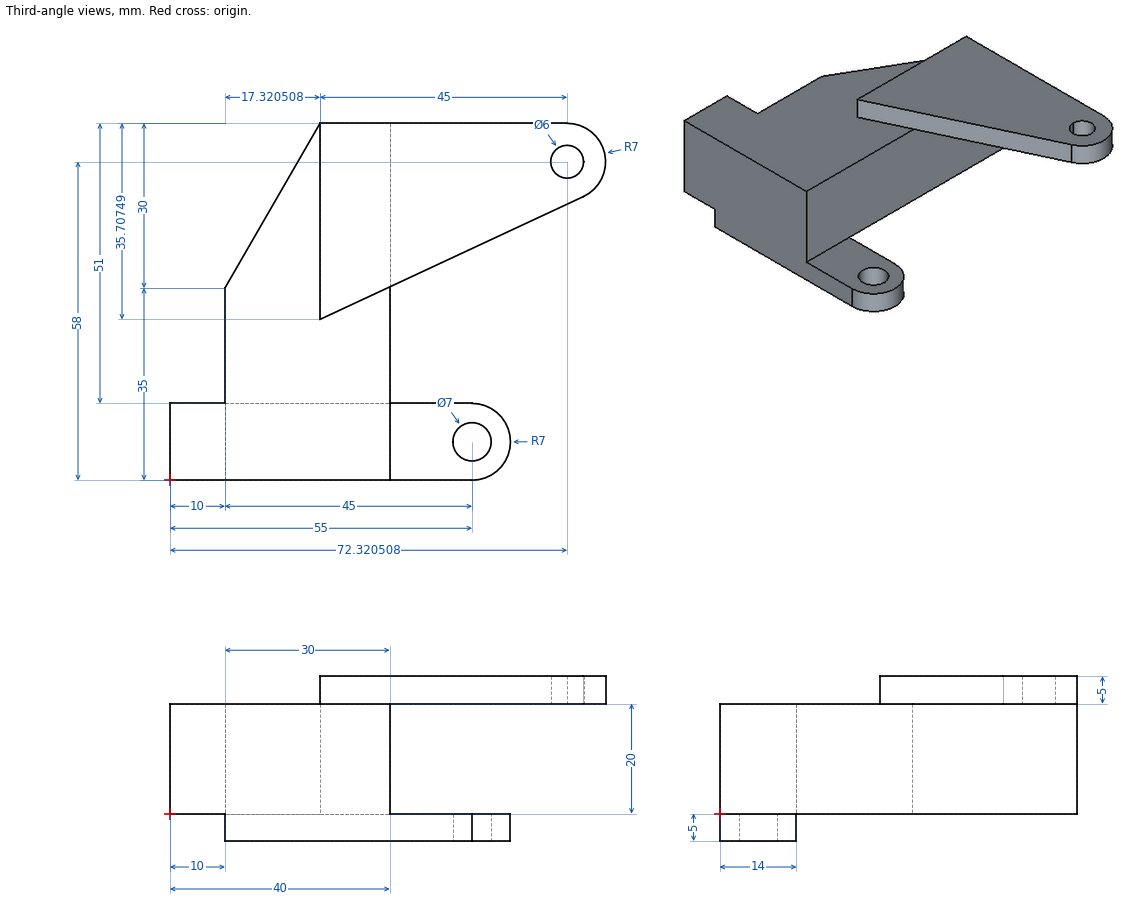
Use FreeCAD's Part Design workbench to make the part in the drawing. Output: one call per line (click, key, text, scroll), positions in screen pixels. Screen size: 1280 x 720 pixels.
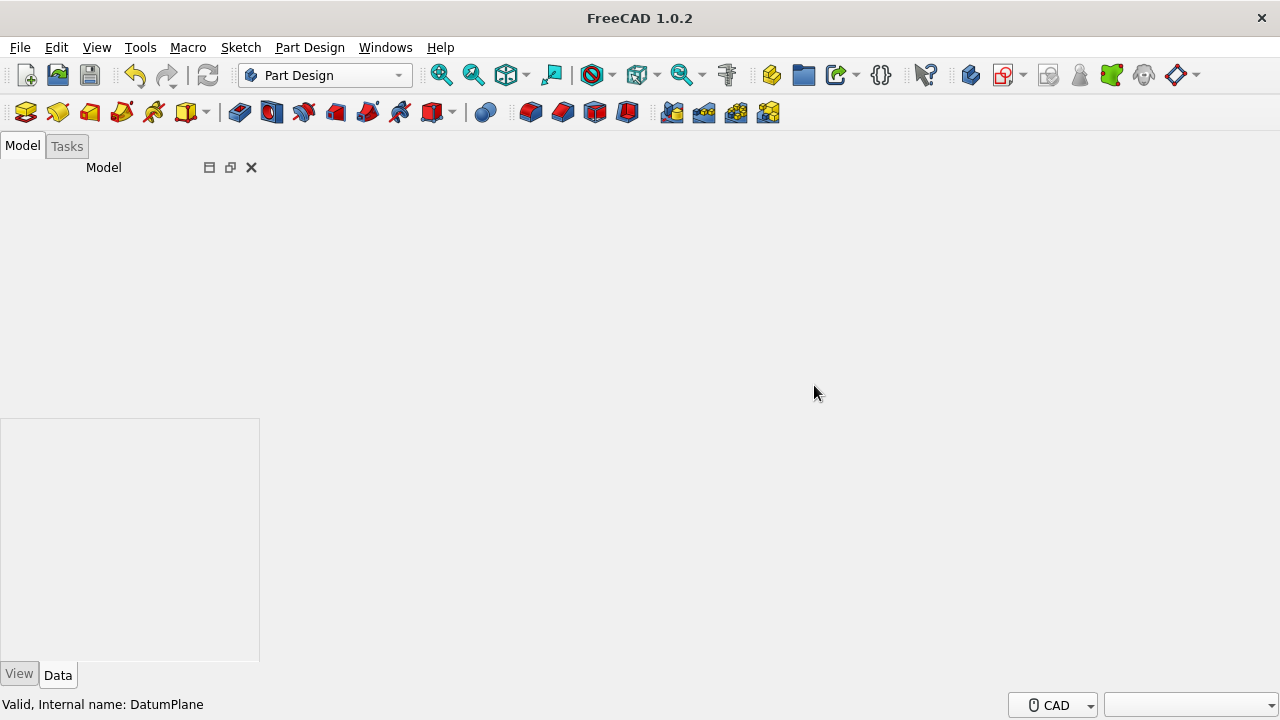
click(26, 76)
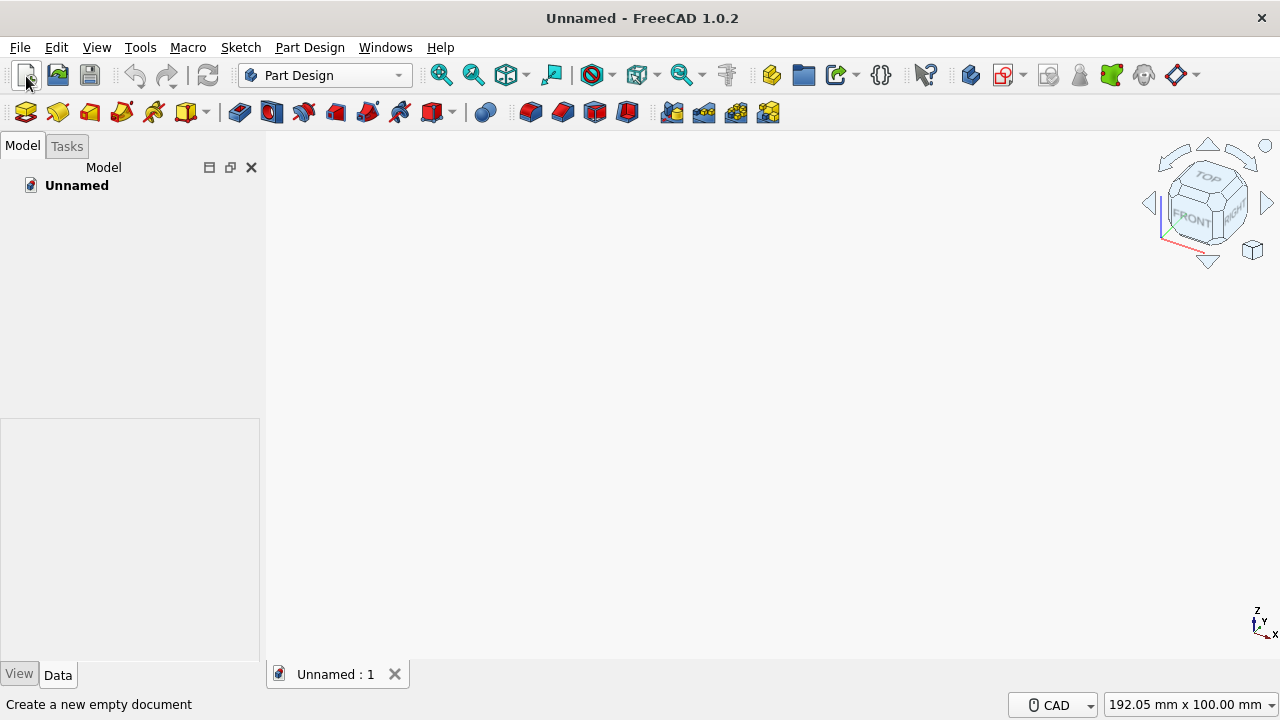
click(1004, 76)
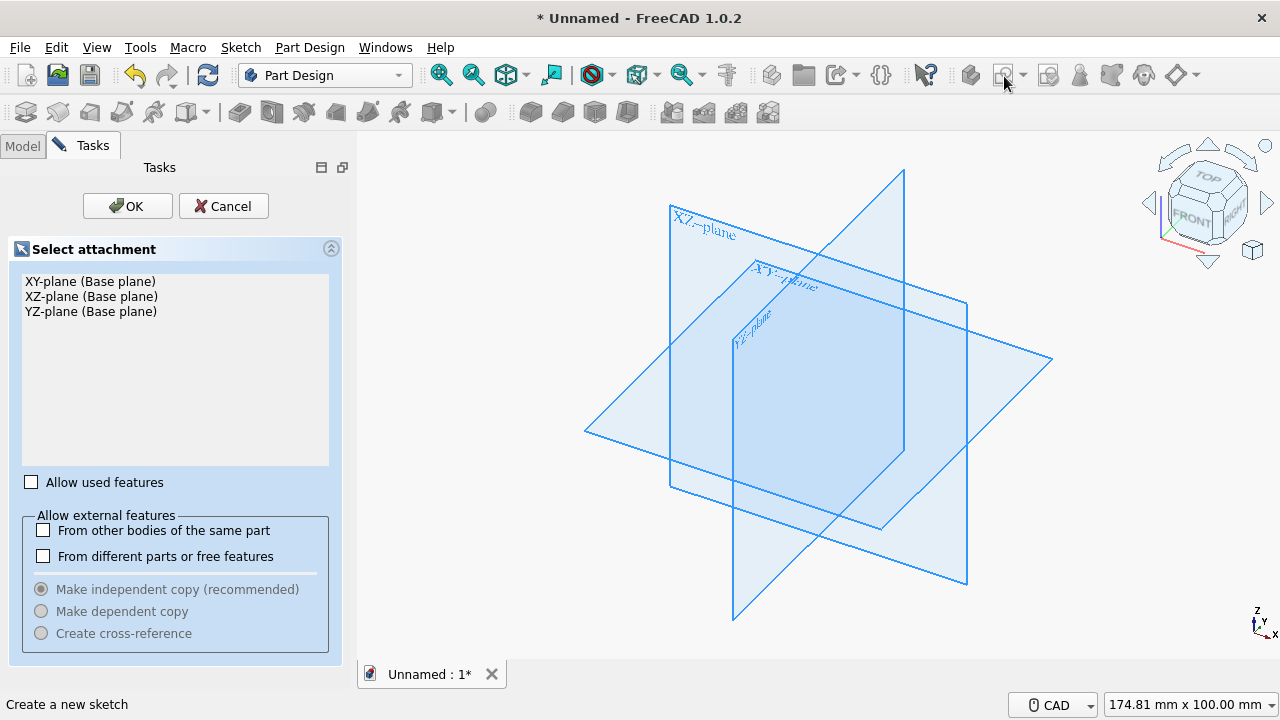
click(82, 296)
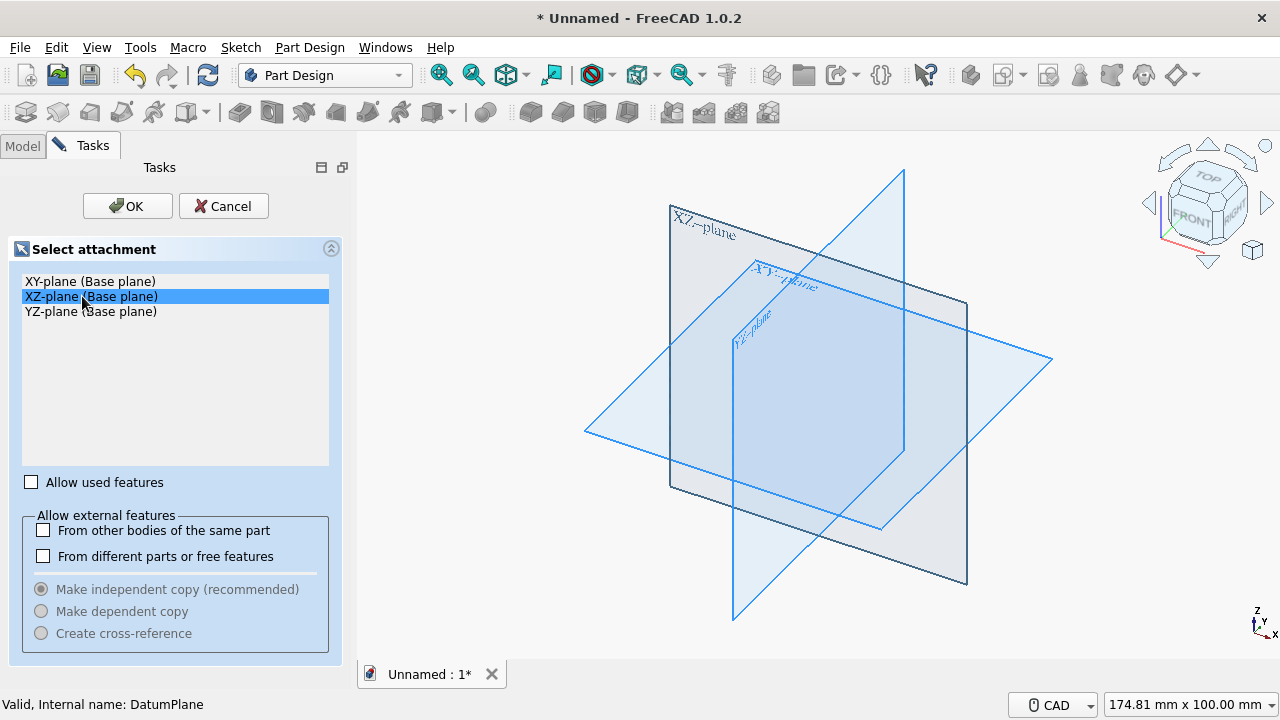
click(128, 206)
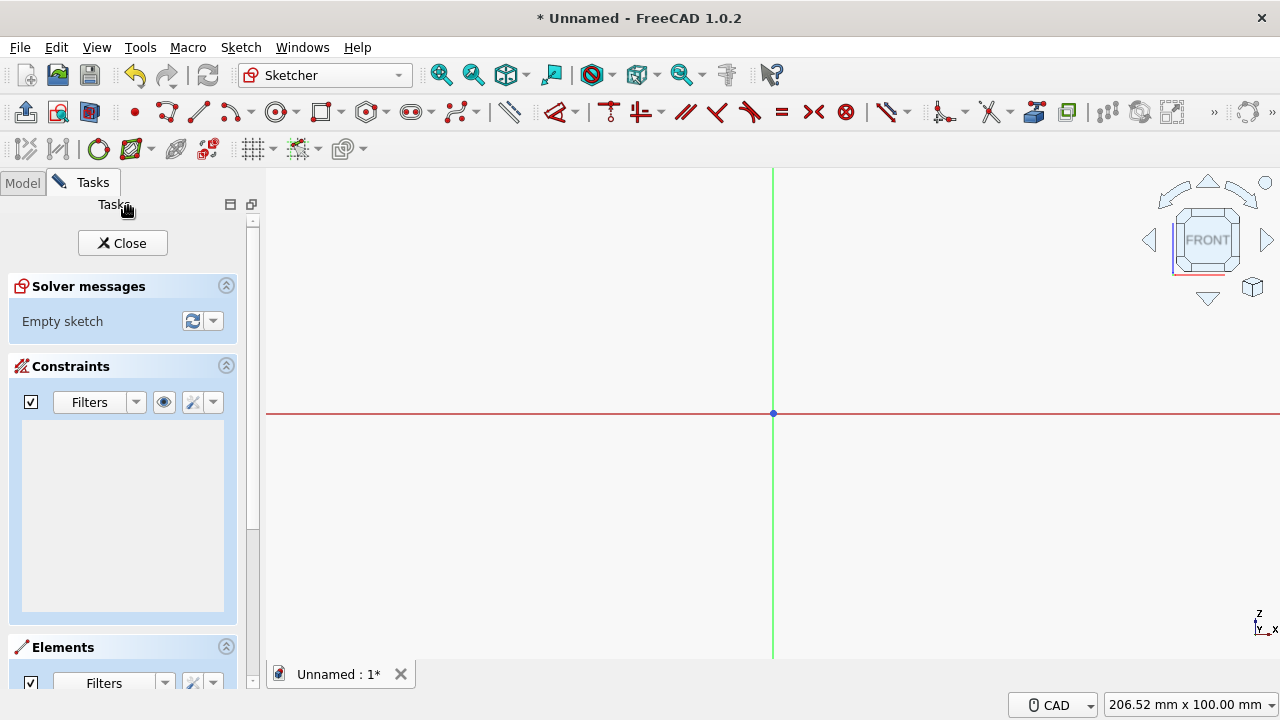
scroll(968, 336, up, 5)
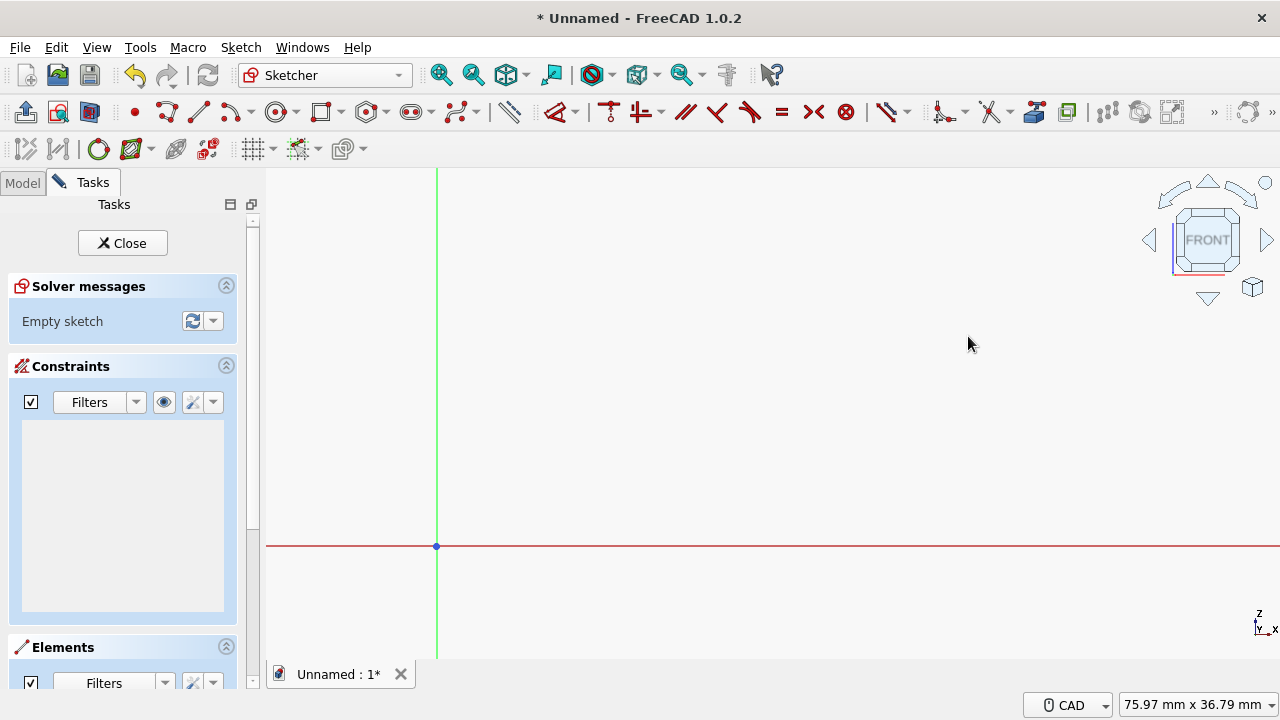
click(322, 112)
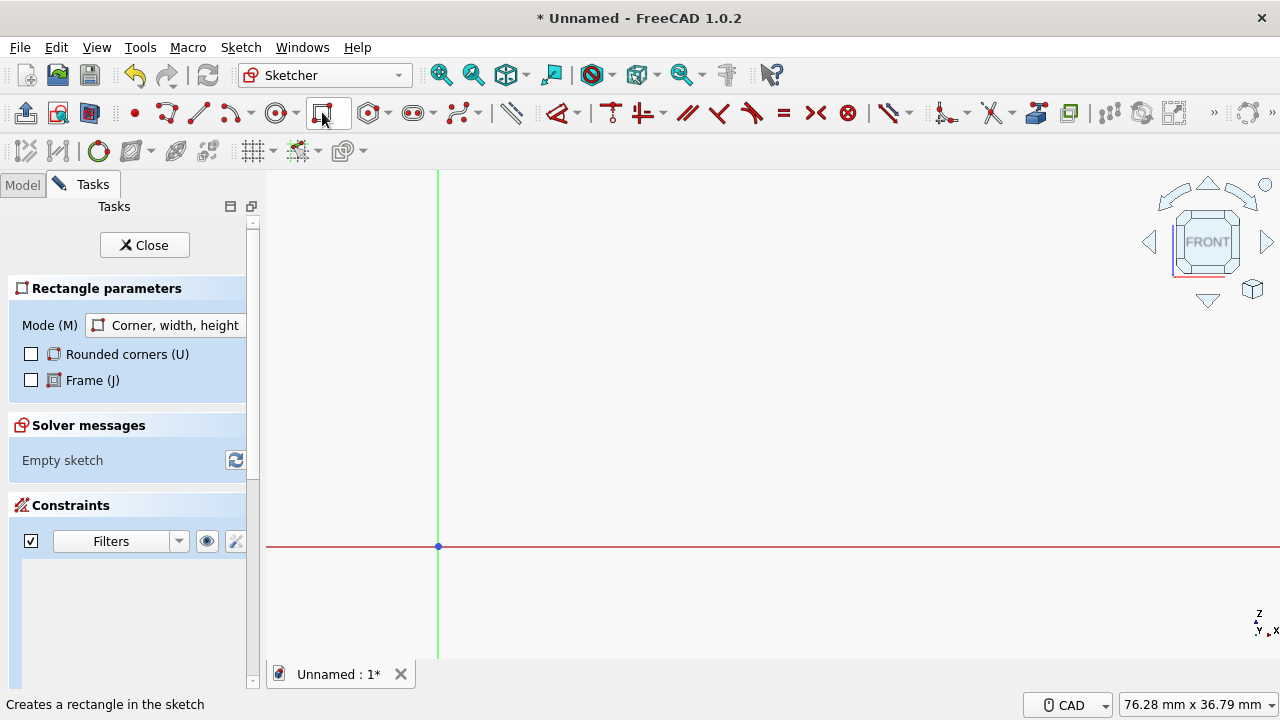
click(438, 547)
click(970, 281)
key(Escape)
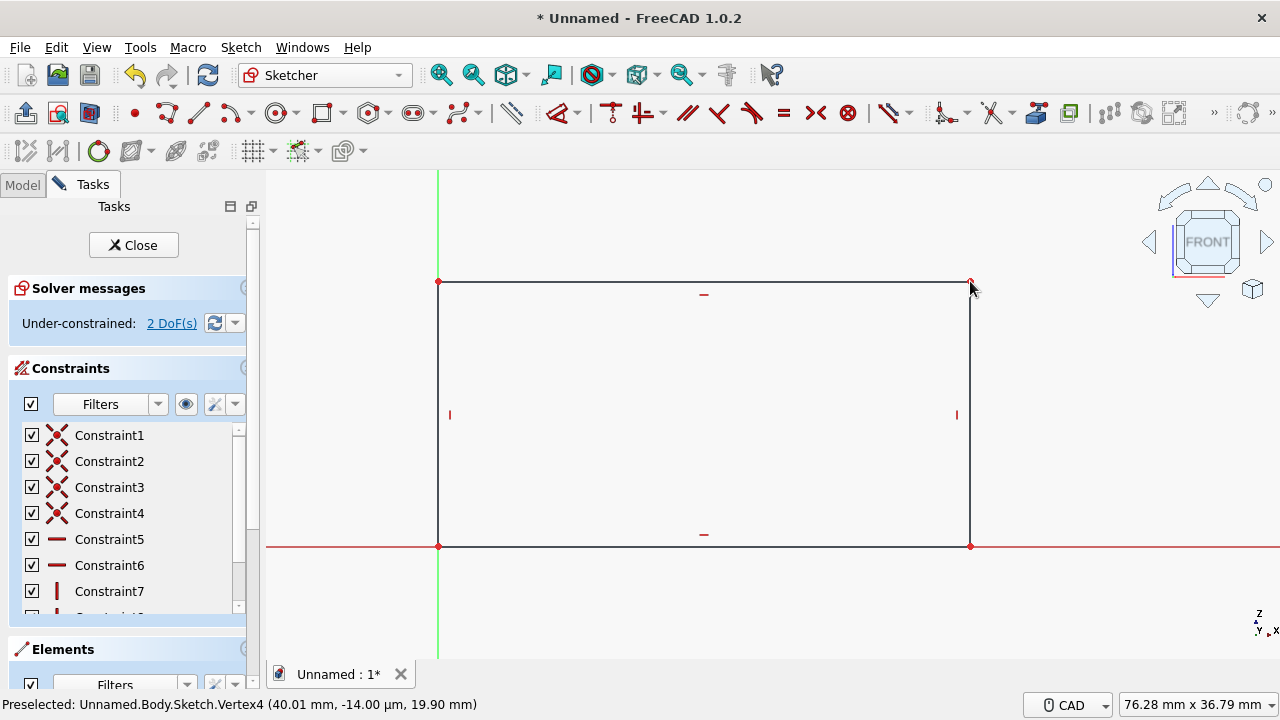
click(558, 114)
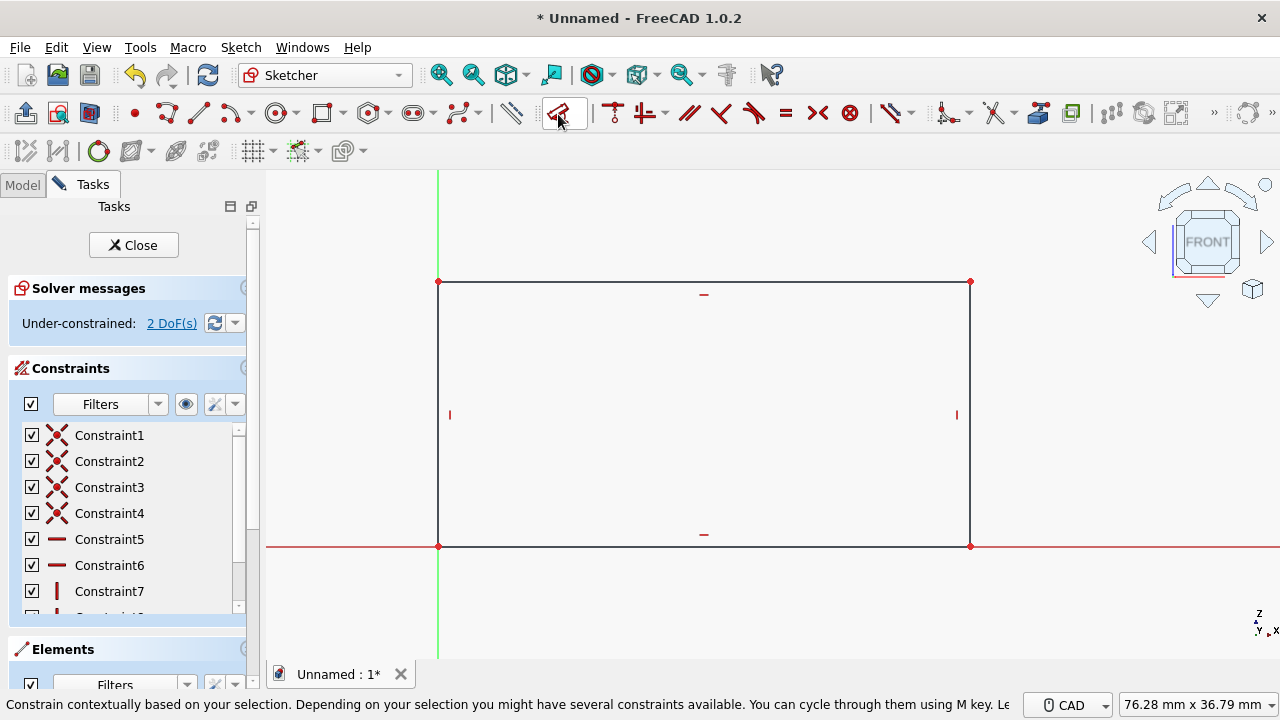
click(598, 547)
click(704, 581)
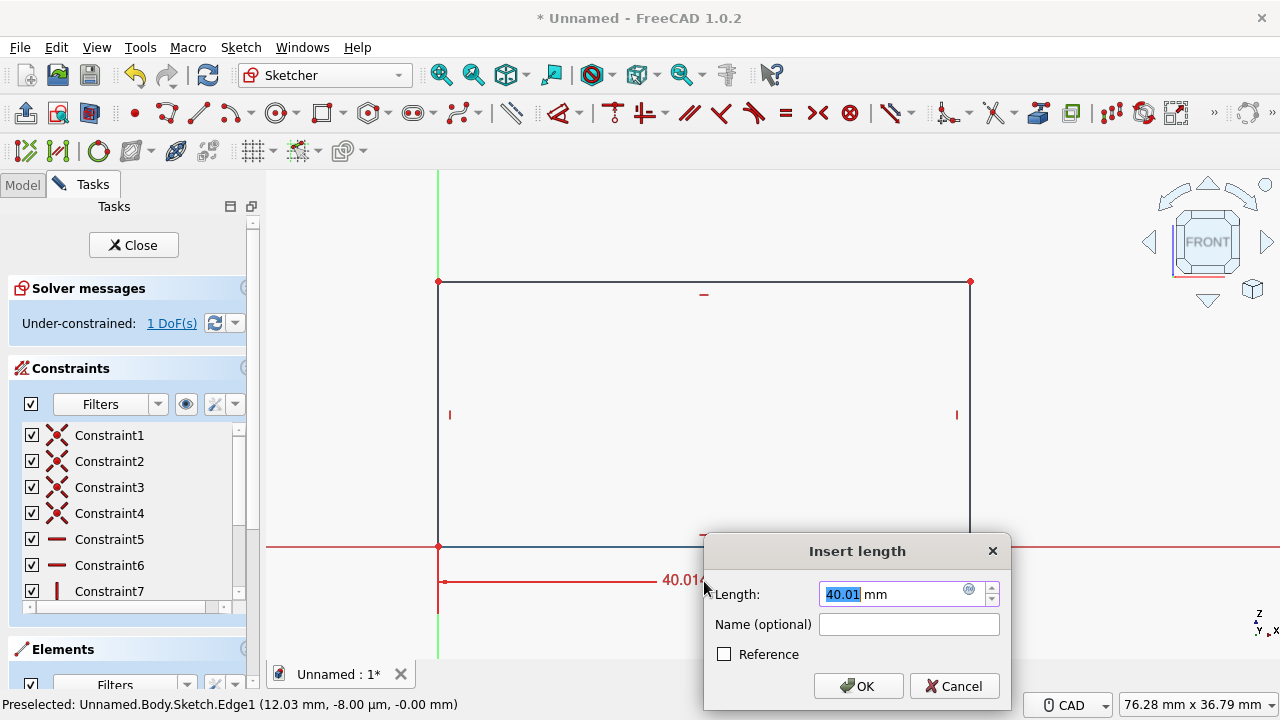
text(40)
key(Return)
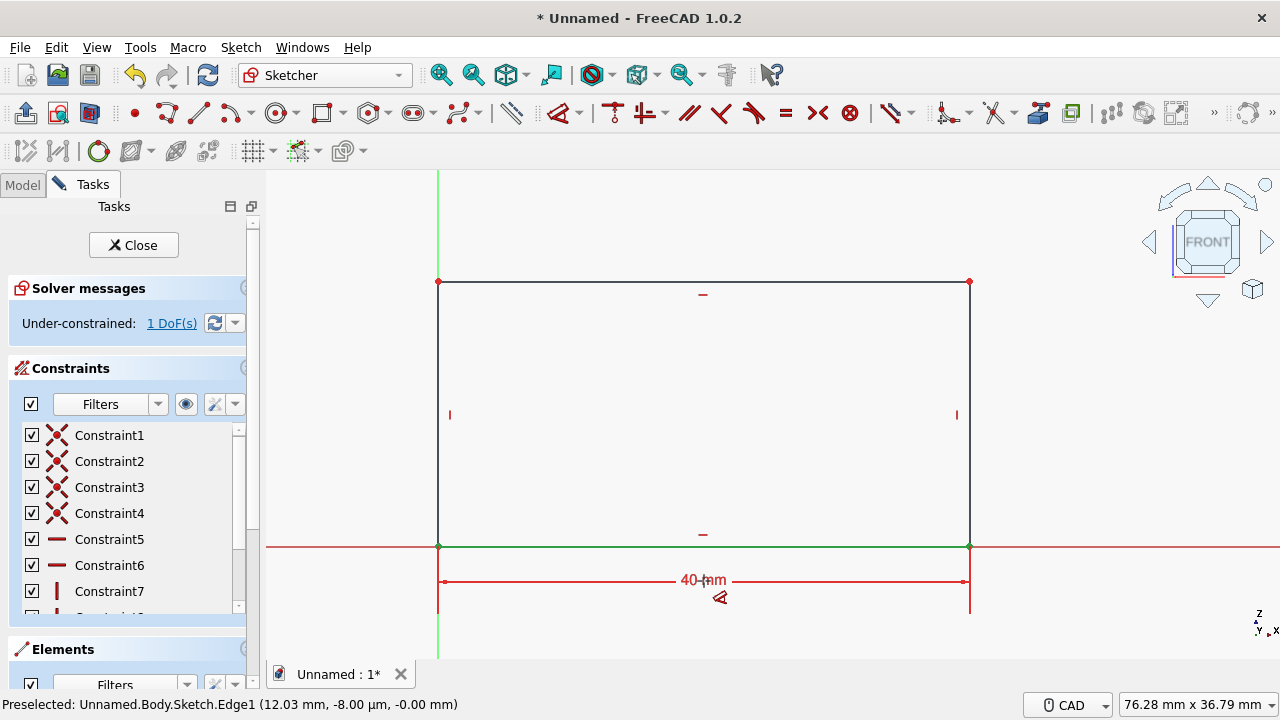
click(970, 467)
click(1004, 414)